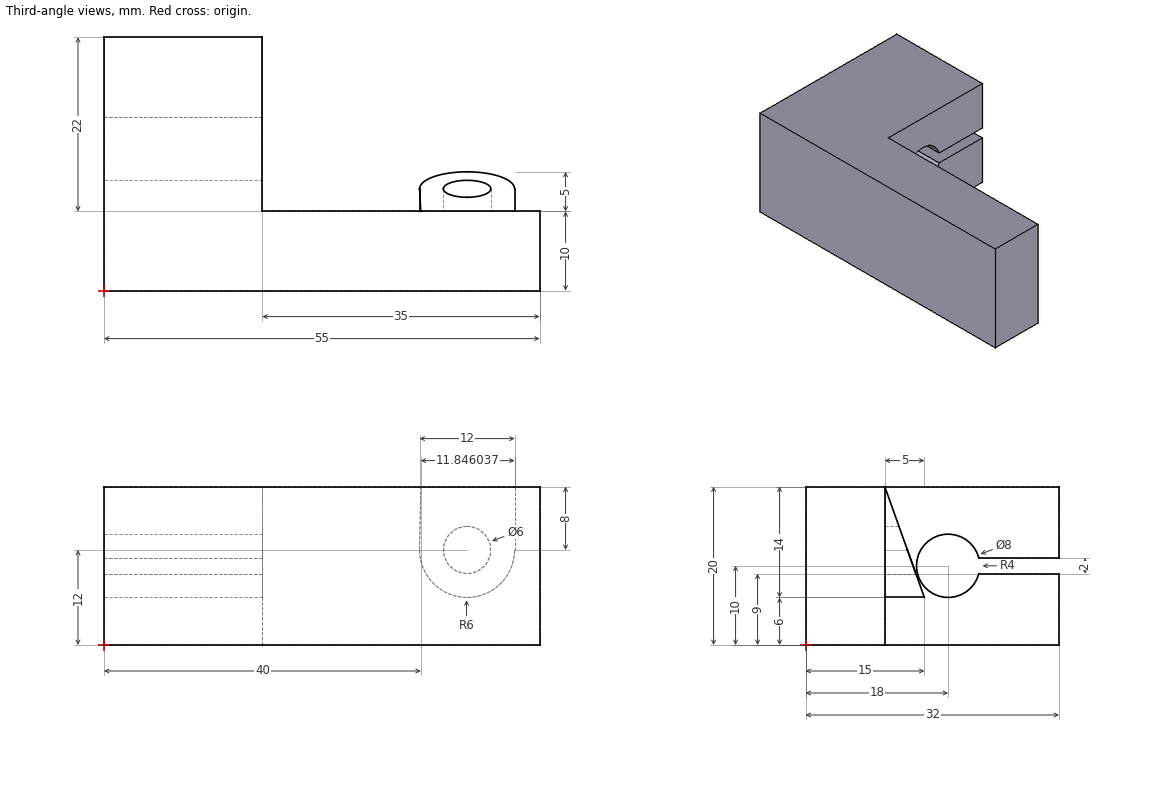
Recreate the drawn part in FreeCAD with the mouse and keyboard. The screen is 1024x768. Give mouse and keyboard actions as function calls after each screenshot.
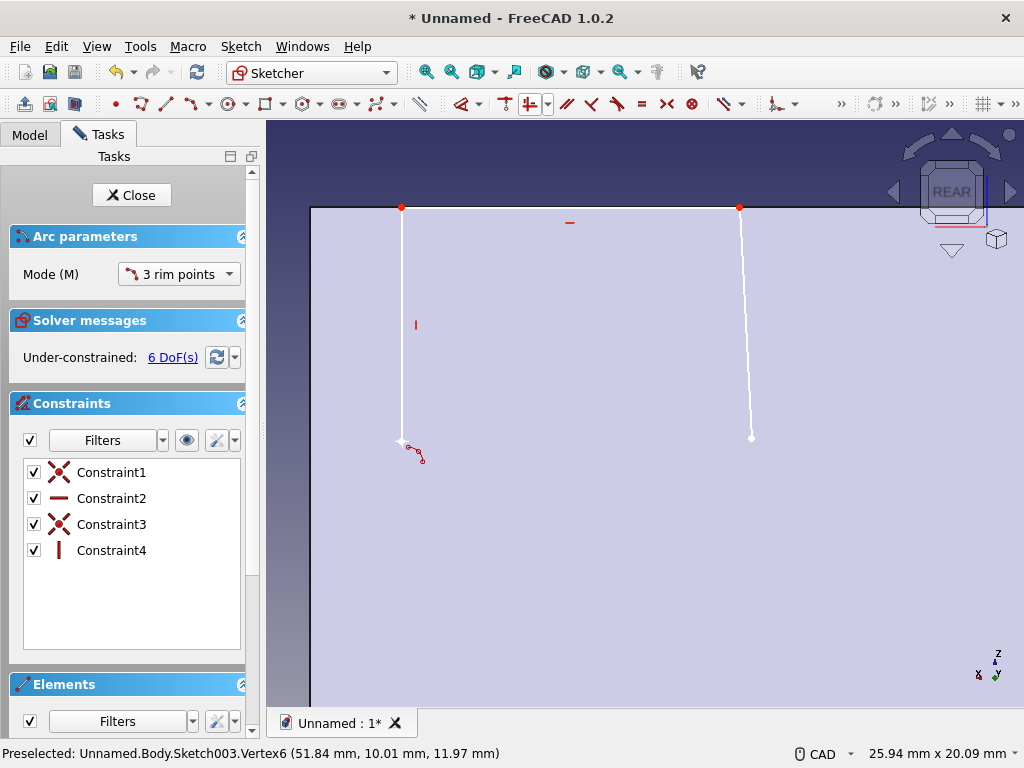
click(402, 442)
click(752, 439)
click(579, 616)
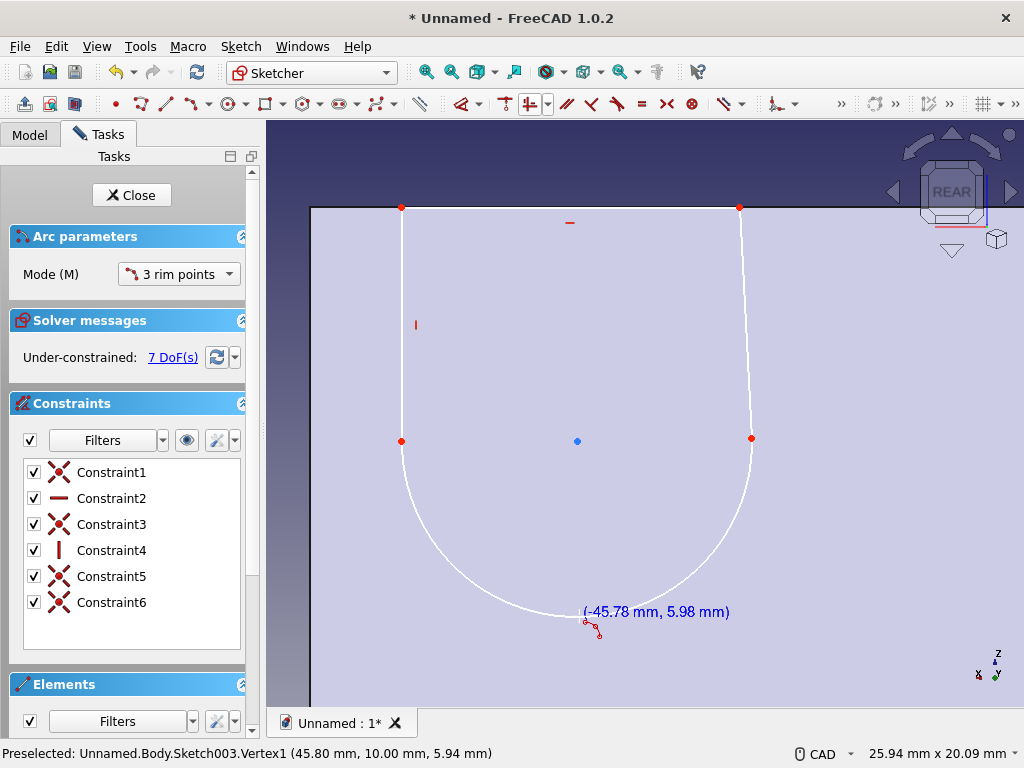
click(228, 104)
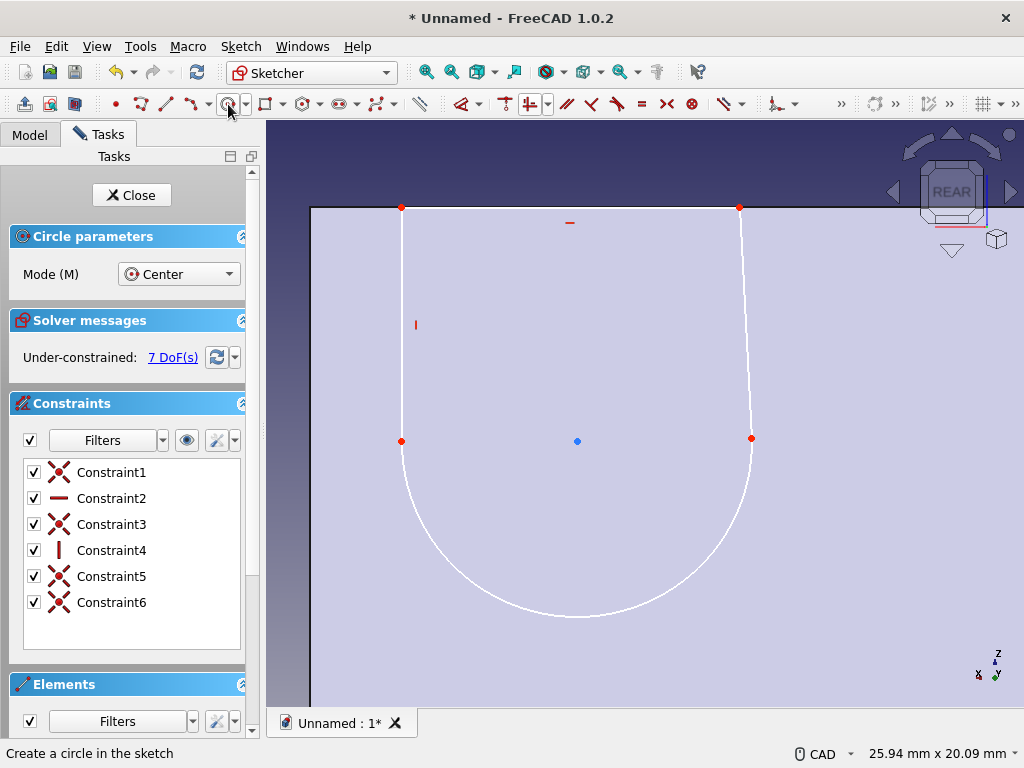
click(577, 441)
move(639, 379)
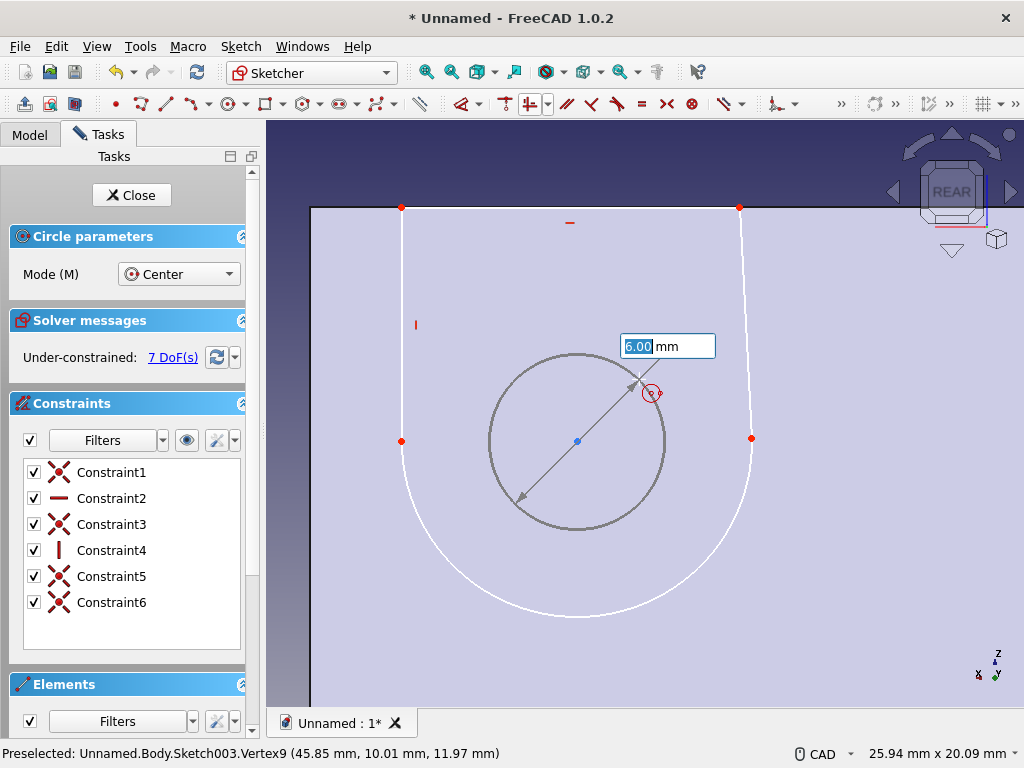
text(6)
key(Return)
key(Escape)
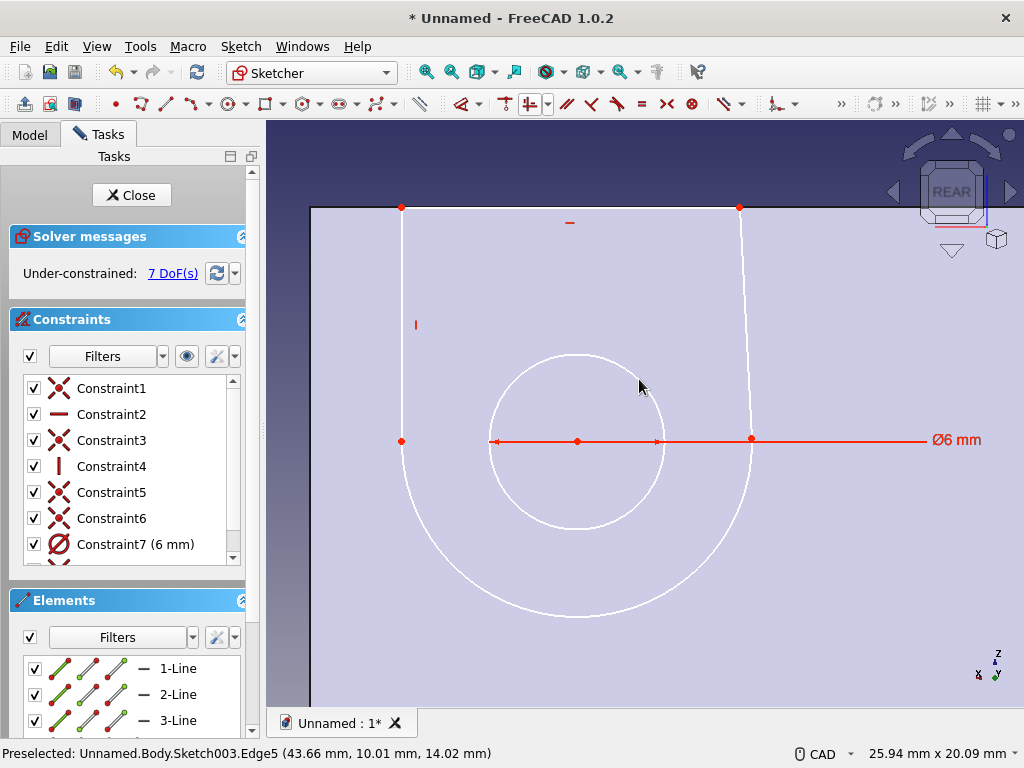
click(748, 370)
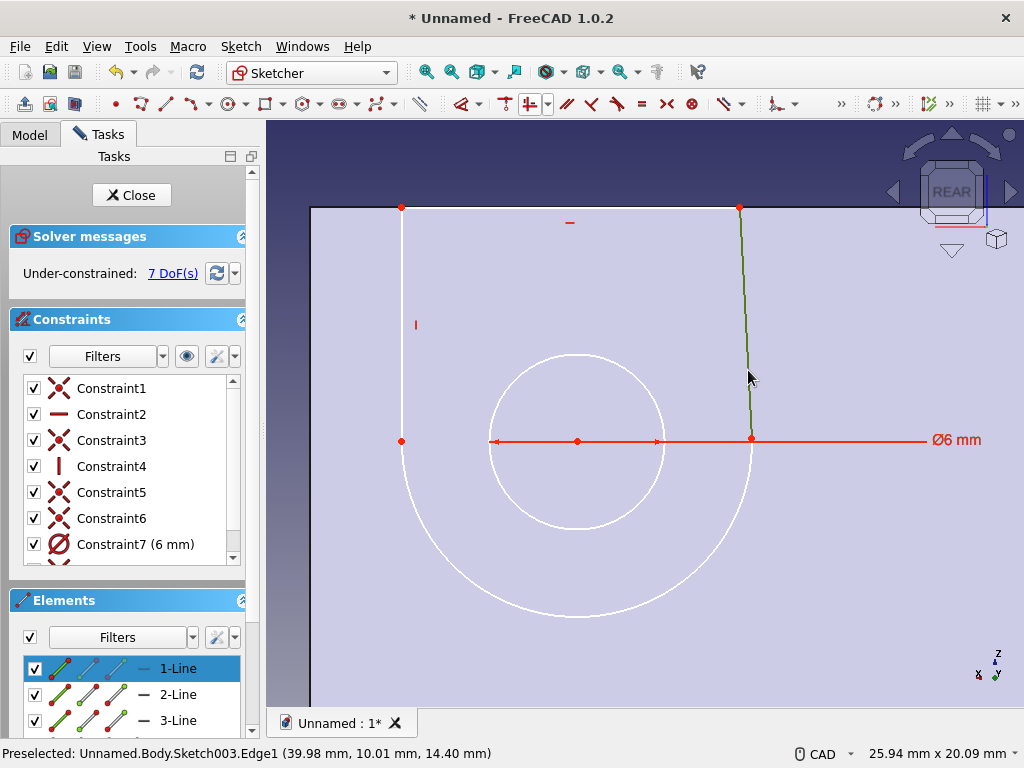
click(475, 584)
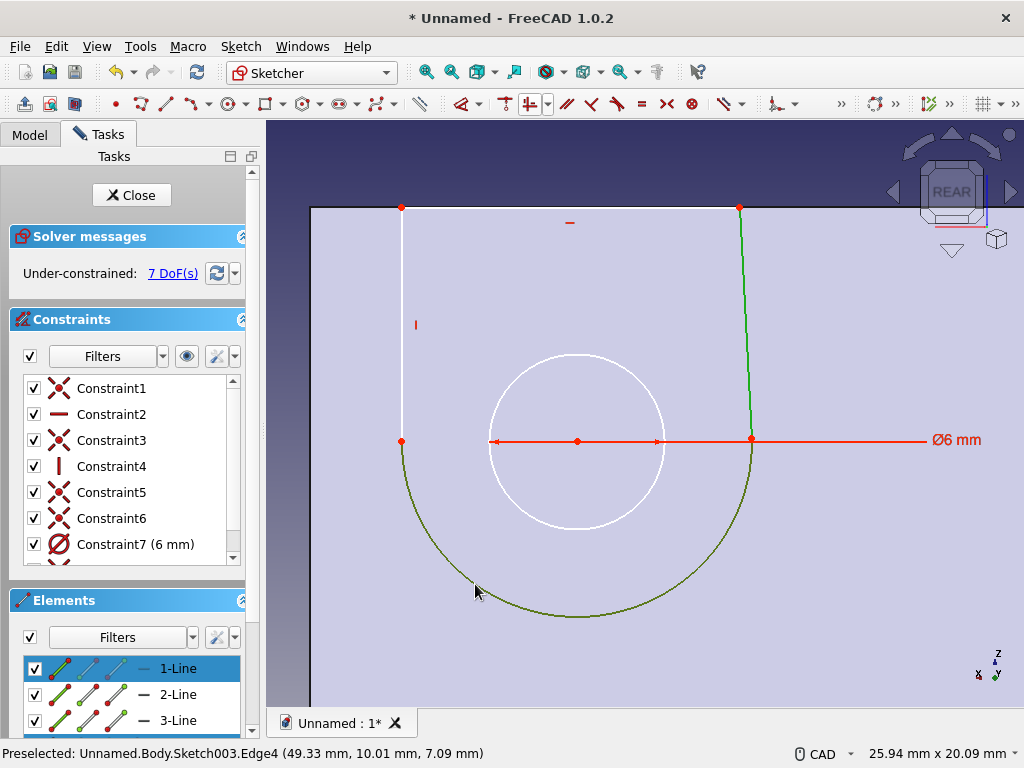
key(t)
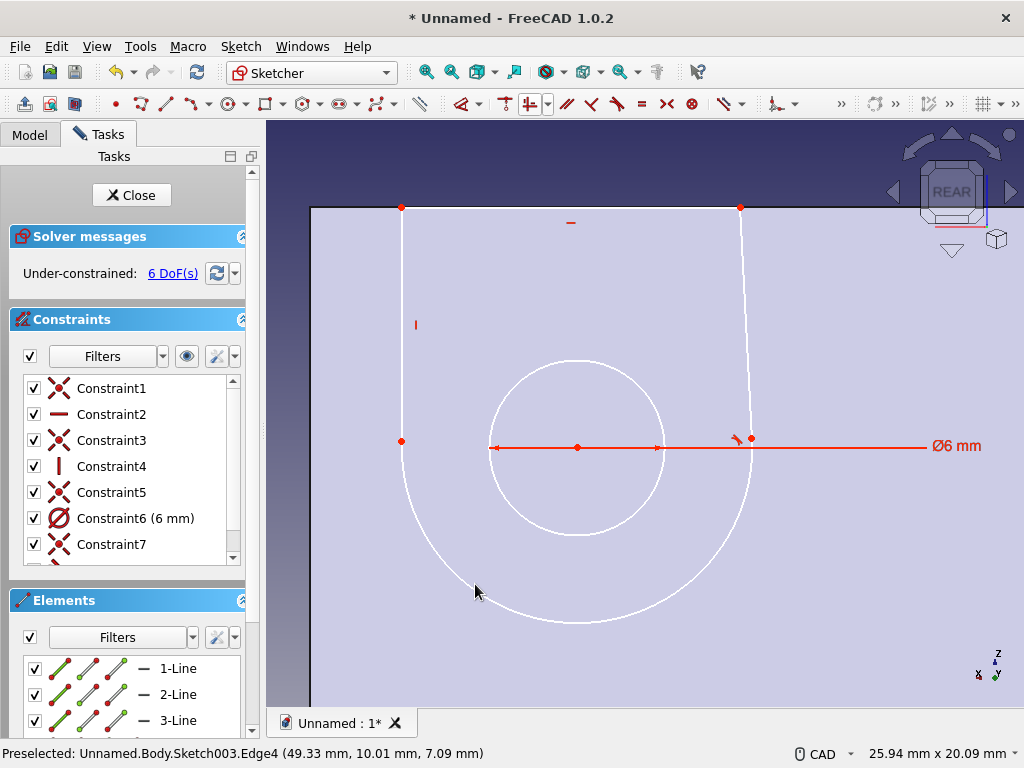
click(402, 278)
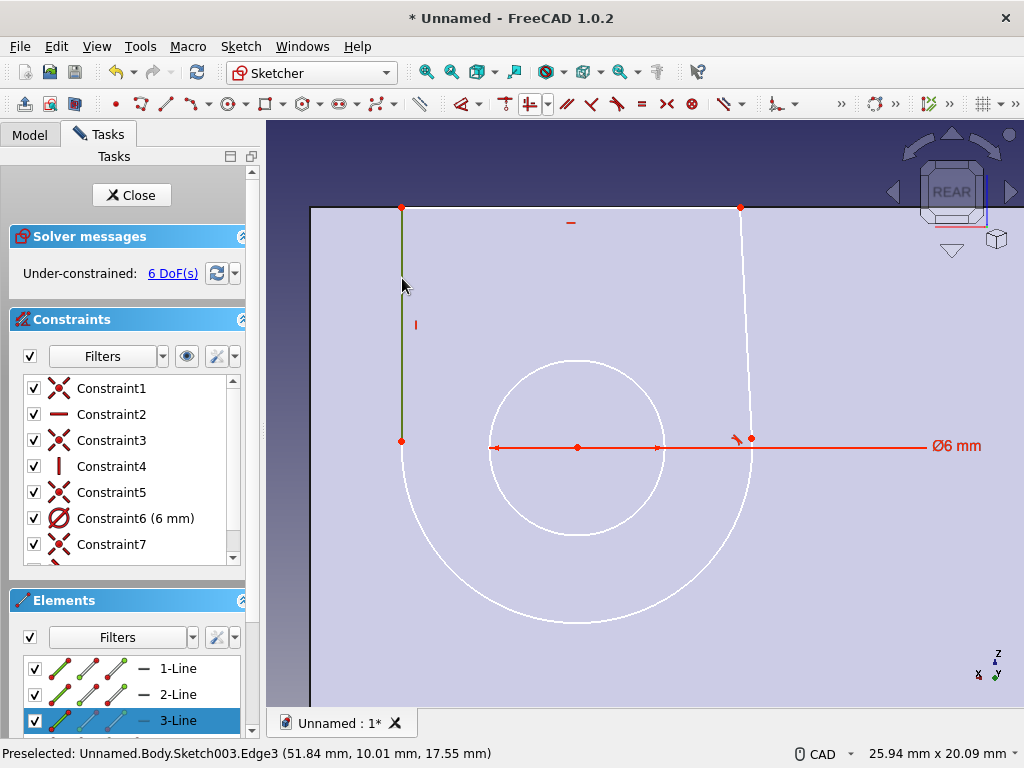
click(473, 589)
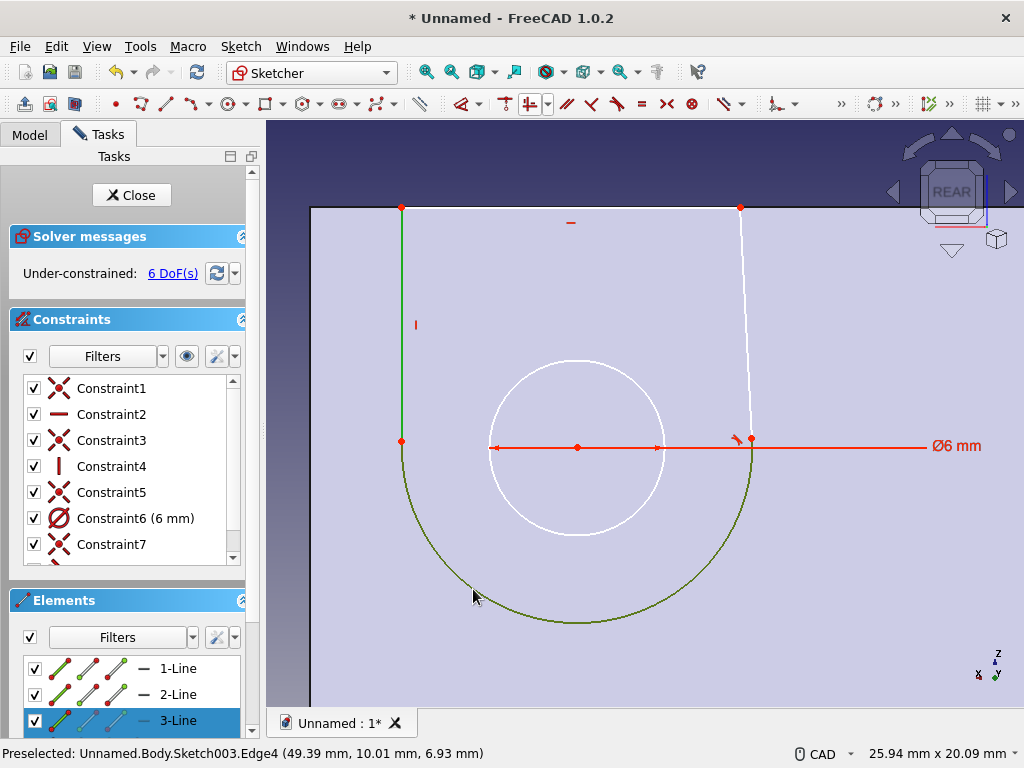
key(t)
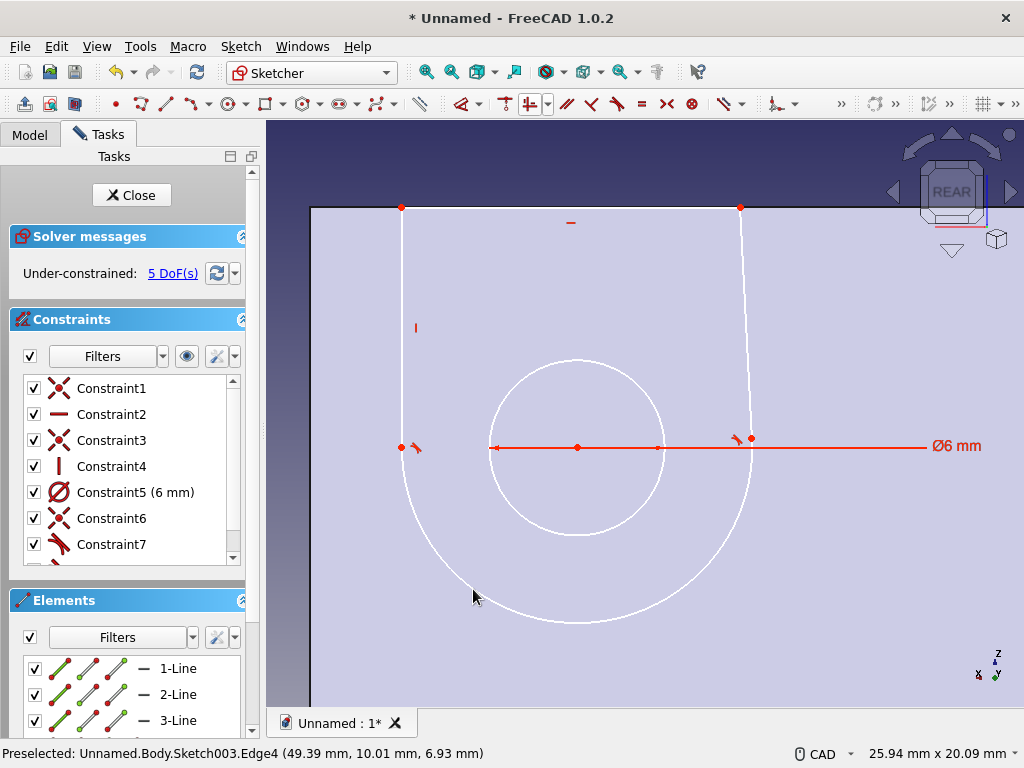
key(d)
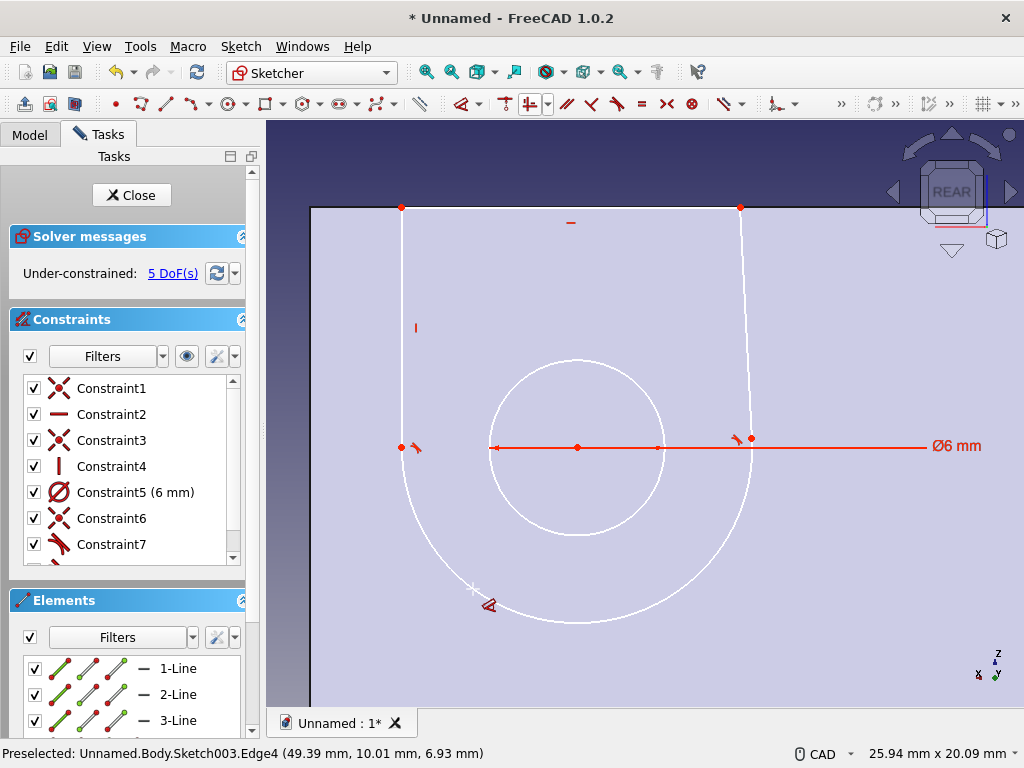
click(476, 591)
click(458, 617)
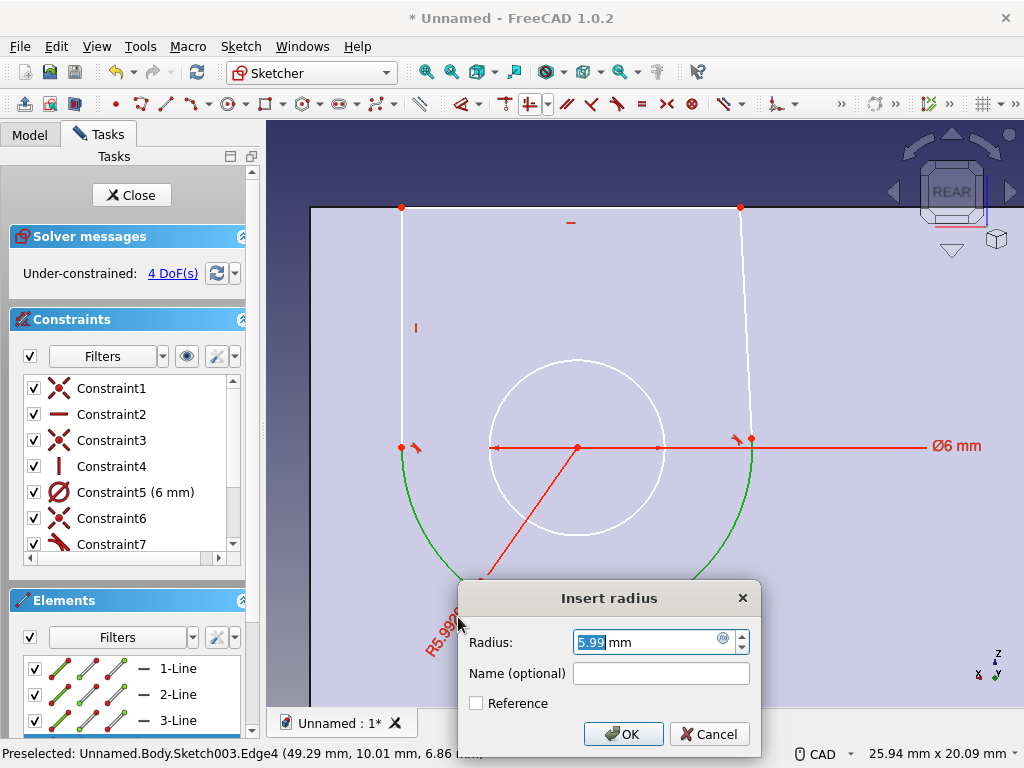
text(6)
key(Return)